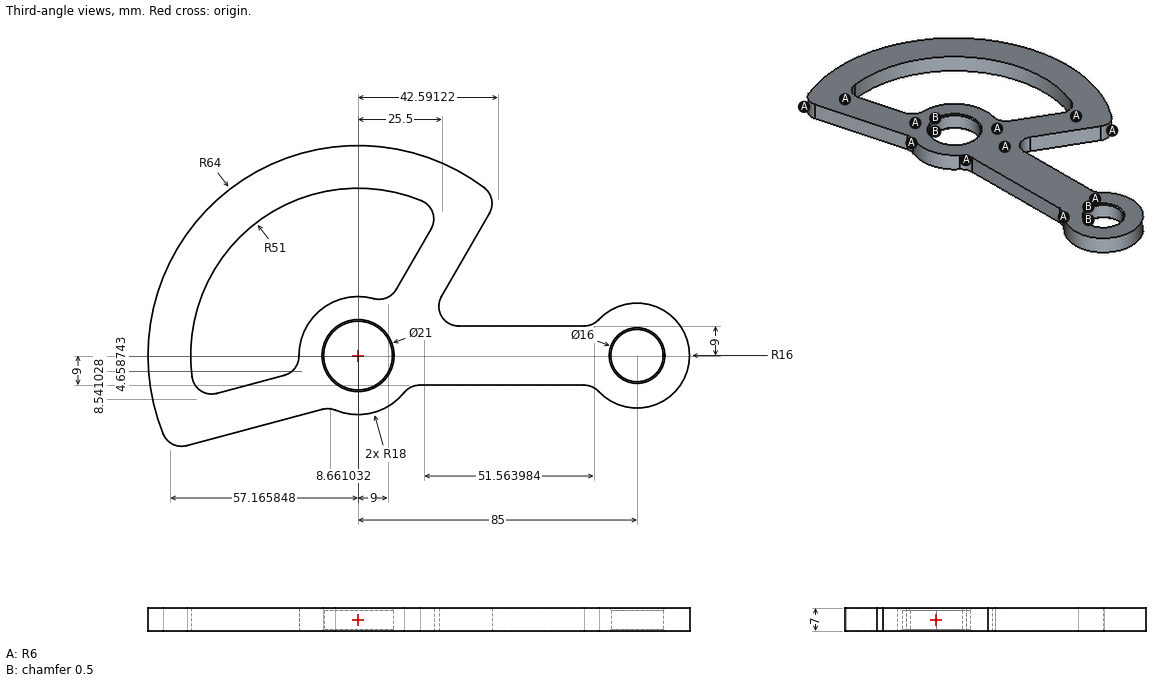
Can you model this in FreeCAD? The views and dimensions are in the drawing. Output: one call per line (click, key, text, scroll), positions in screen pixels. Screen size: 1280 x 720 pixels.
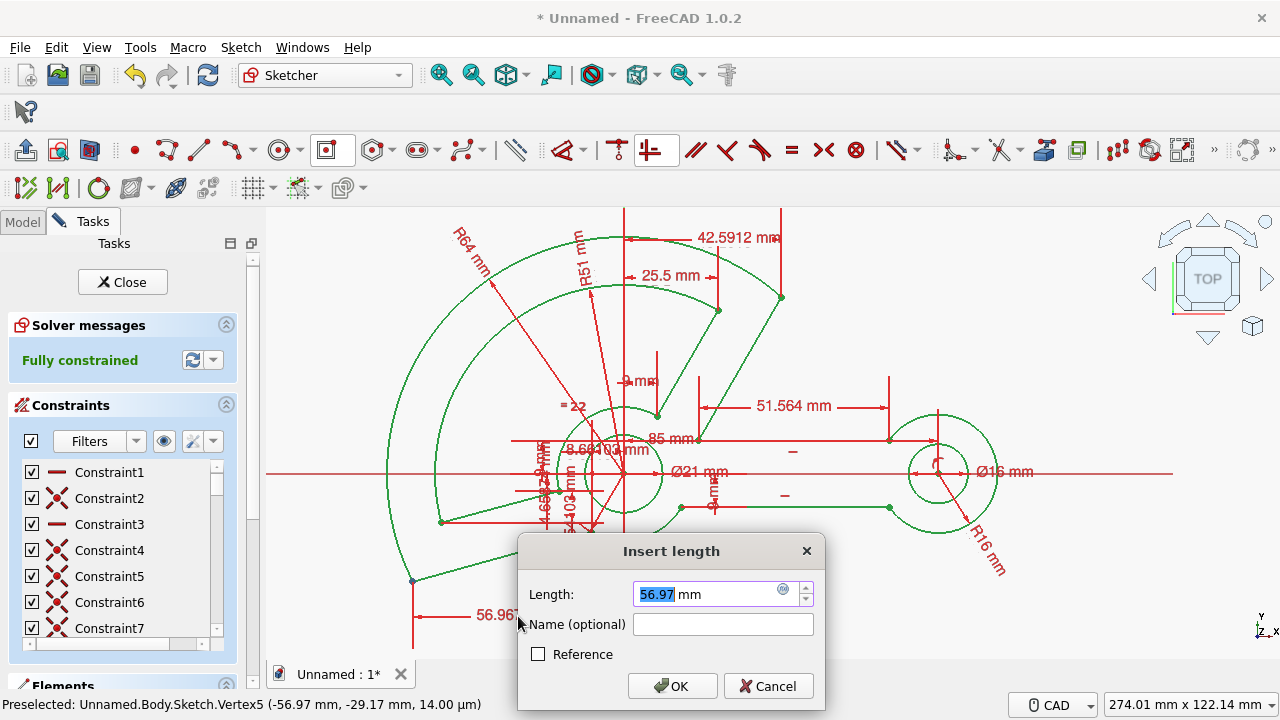
text(57.165848)
key(Return)
key(Escape)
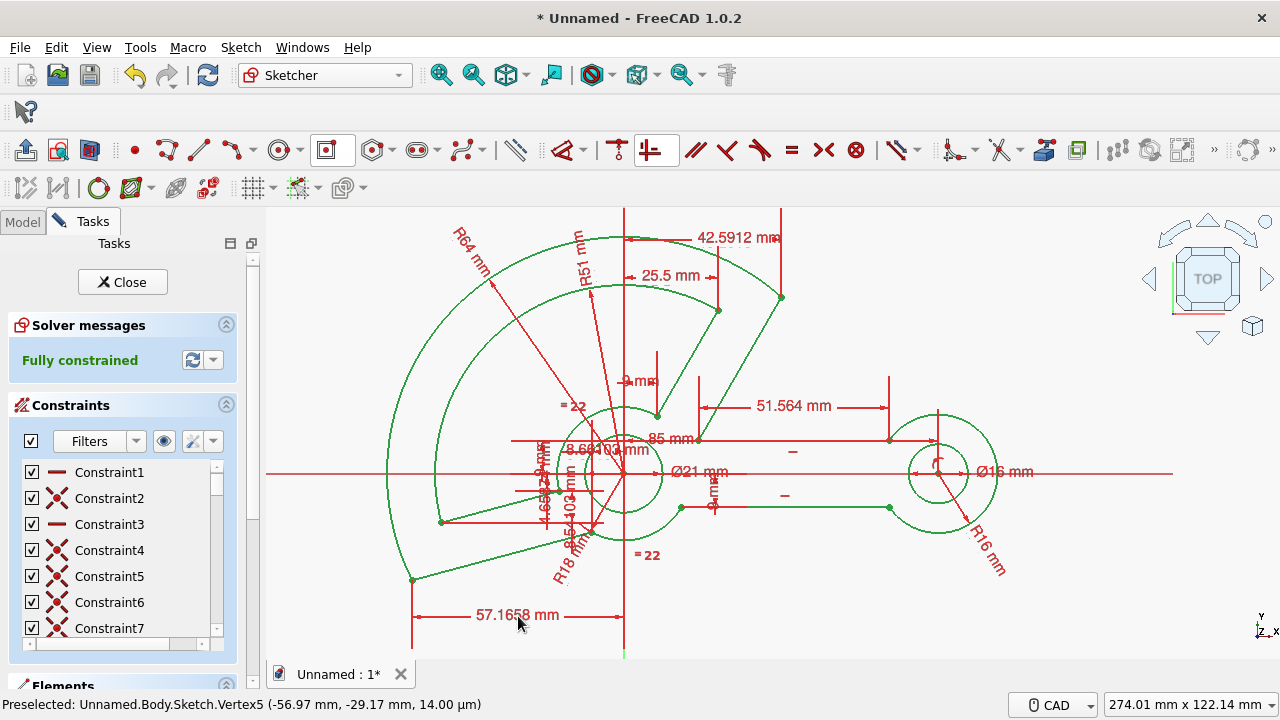
click(123, 282)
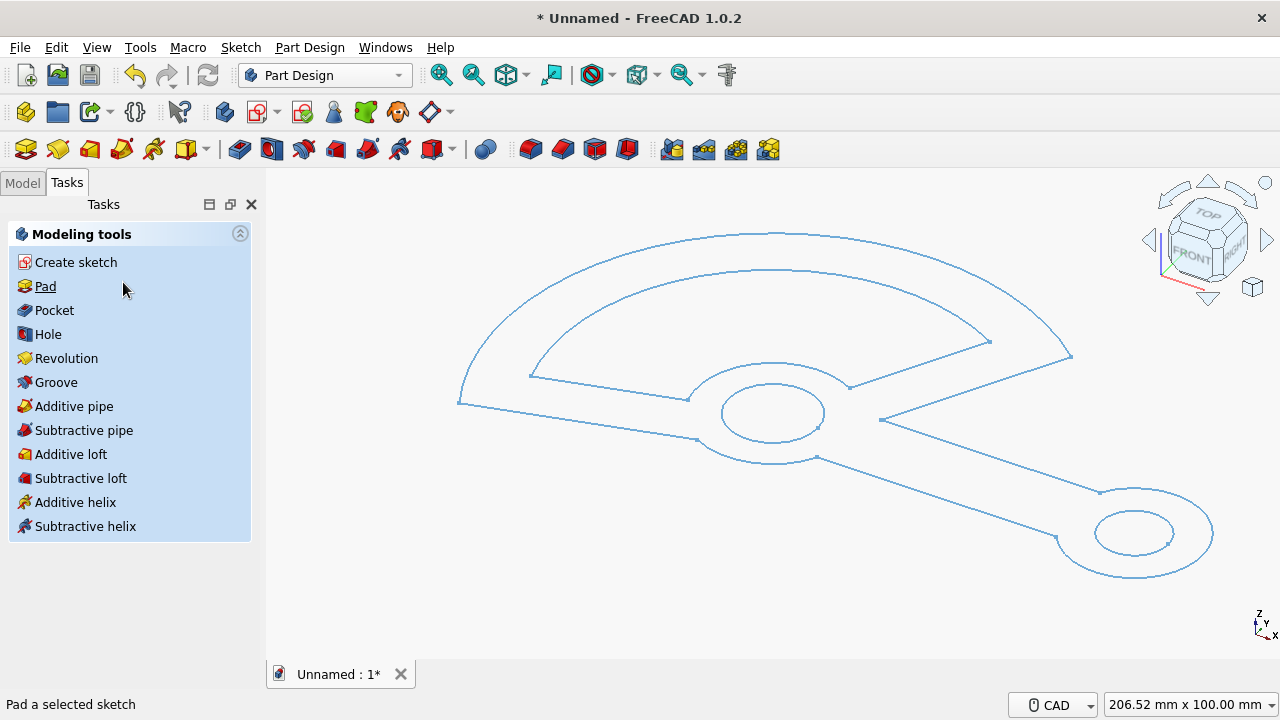
click(26, 150)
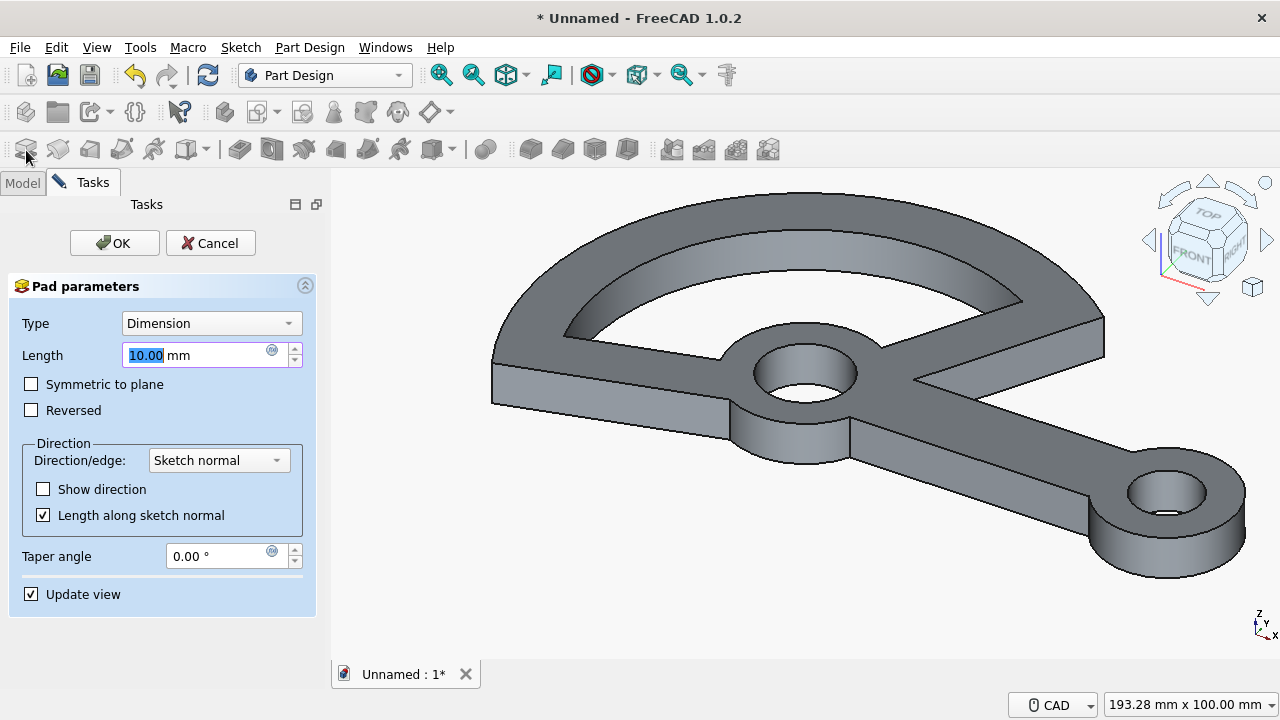
text(7)
key(Tab)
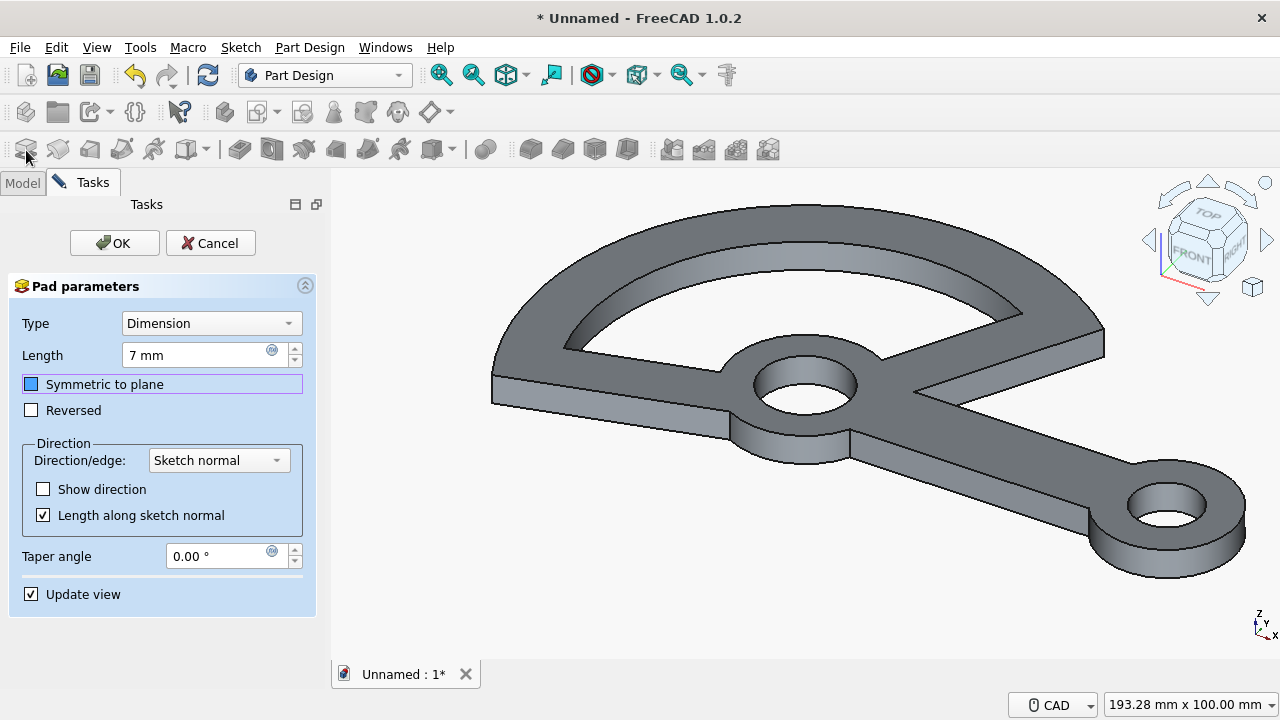
click(30, 384)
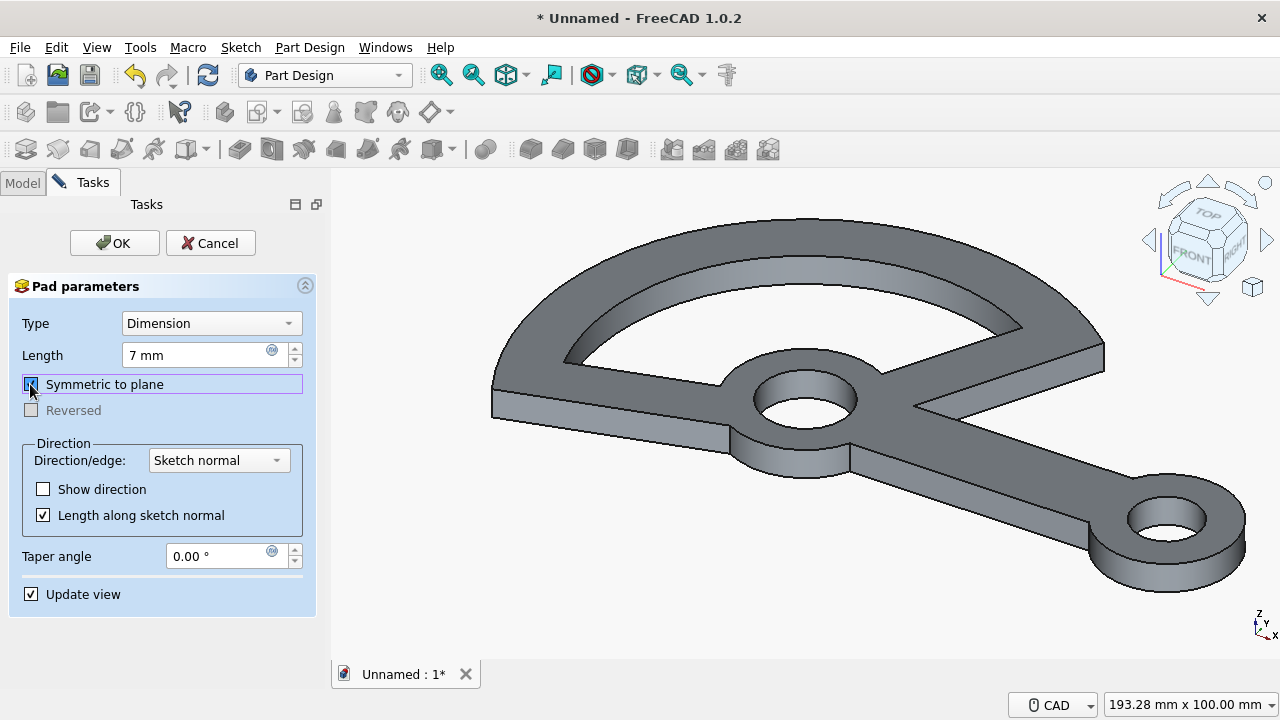
click(115, 243)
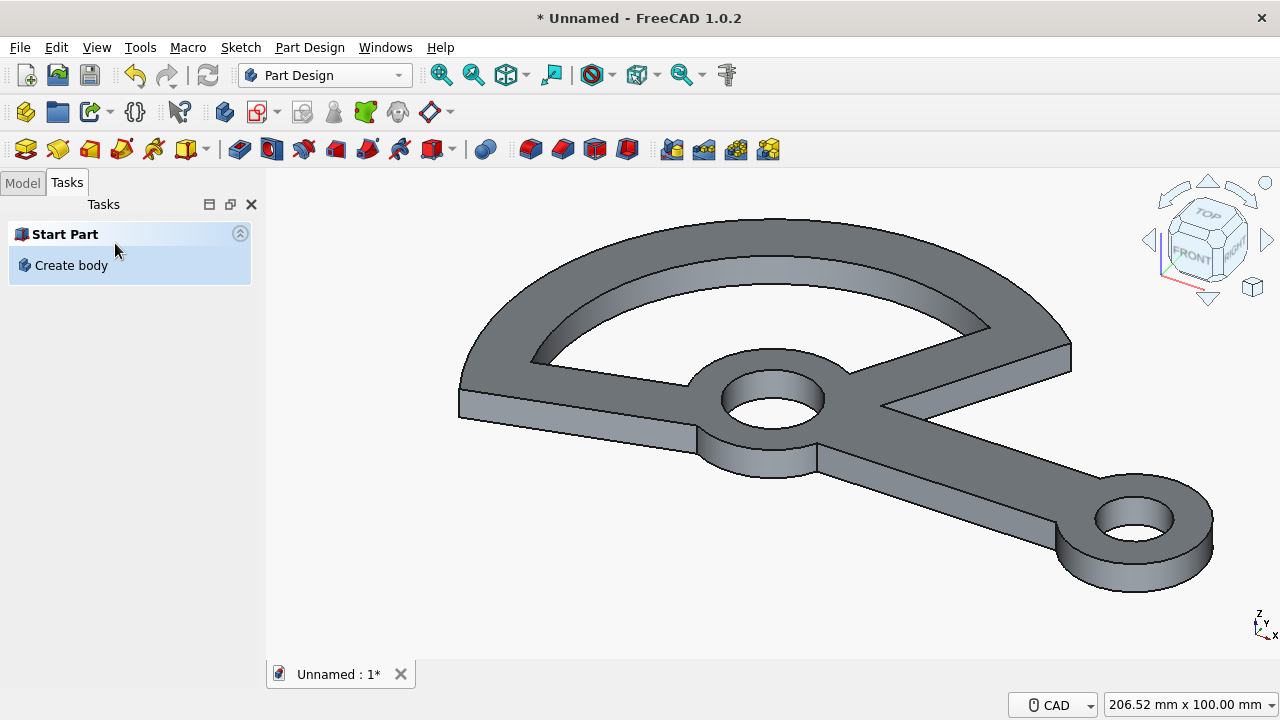
click(442, 76)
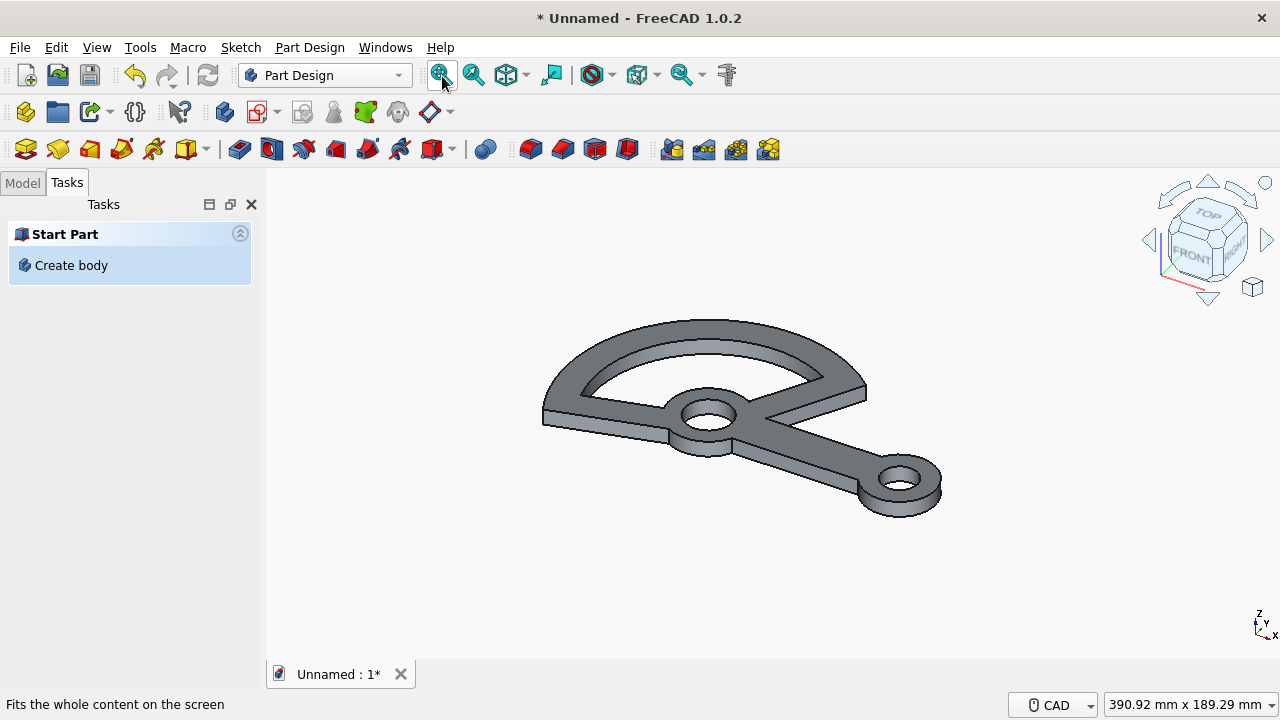
scroll(858, 486, up, 4)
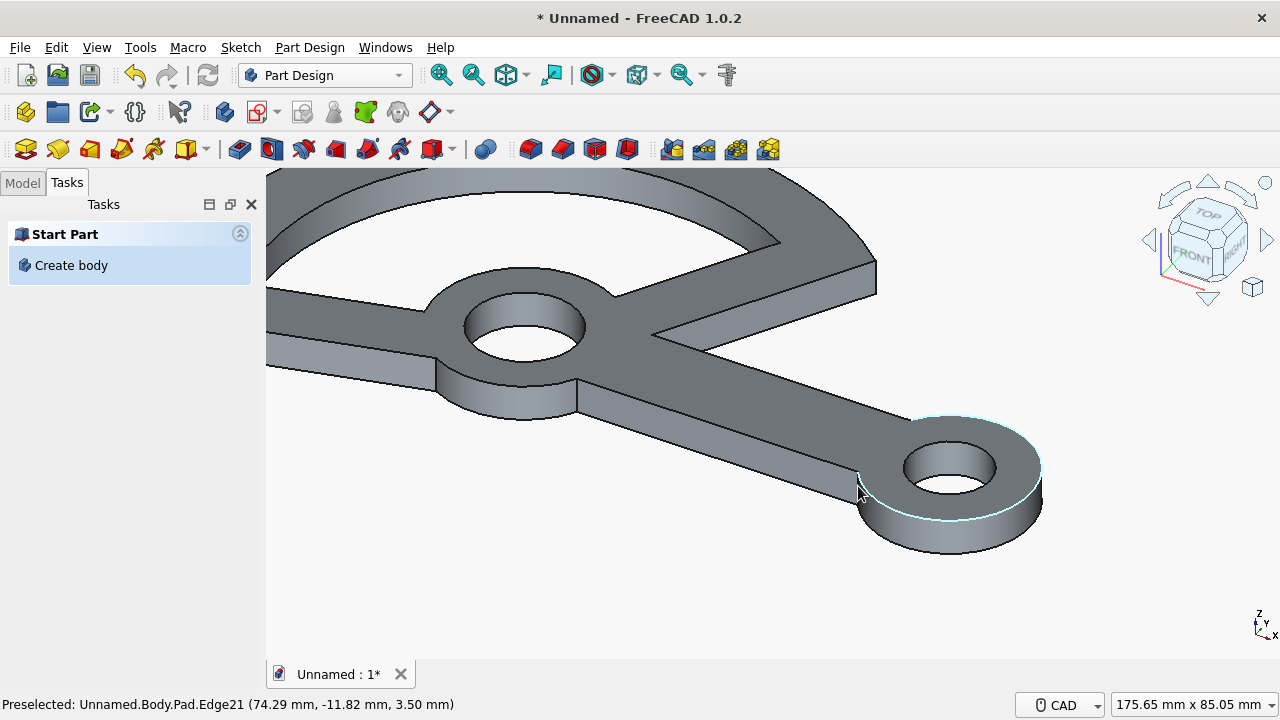
click(442, 76)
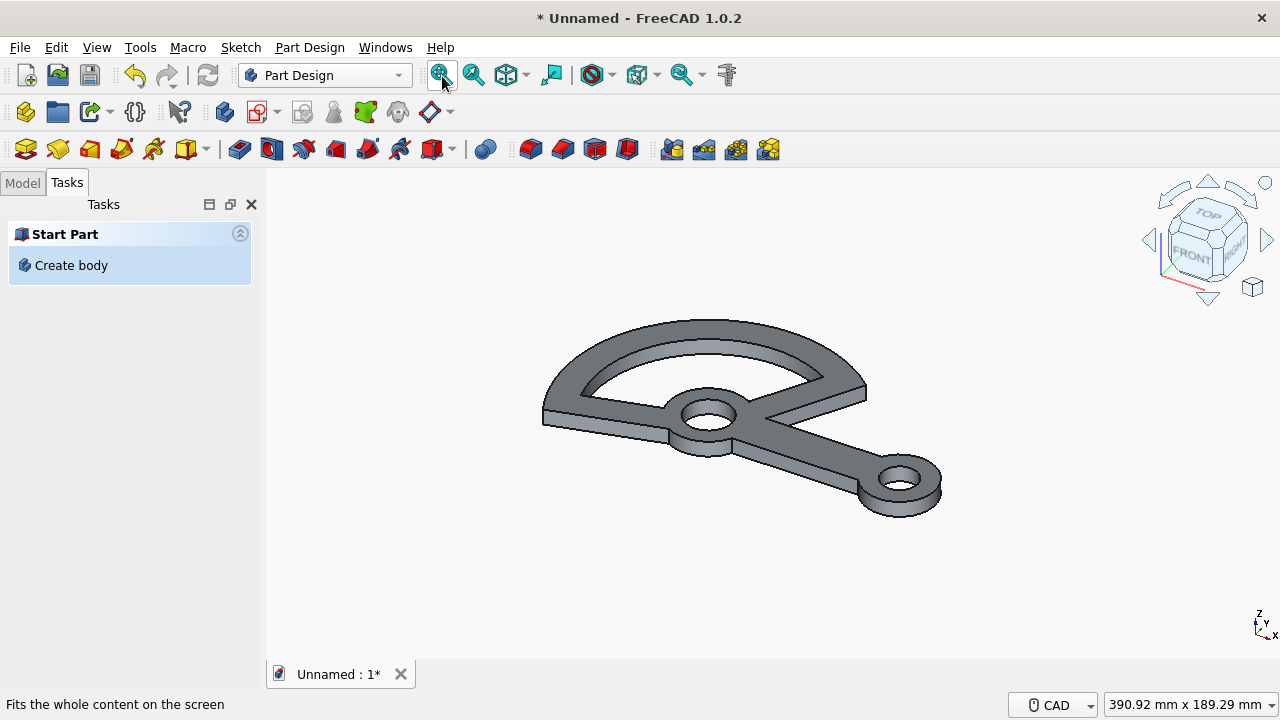
key(0)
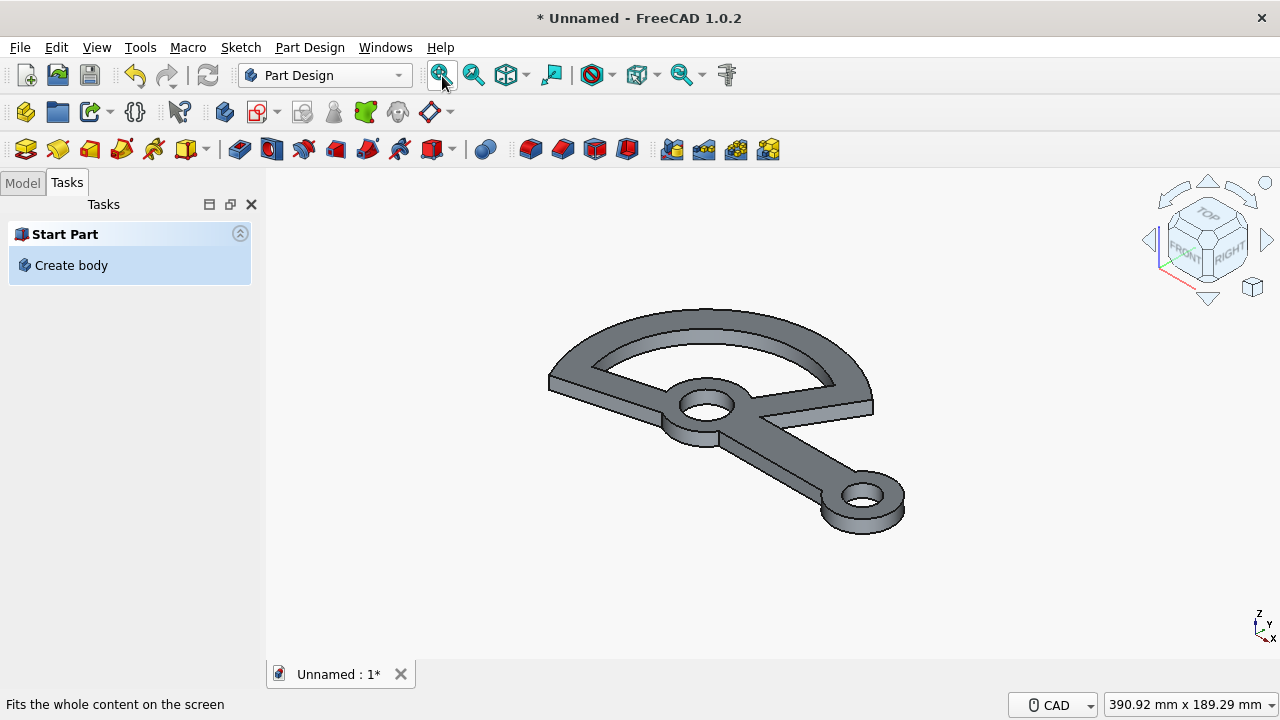
scroll(822, 497, up, 4)